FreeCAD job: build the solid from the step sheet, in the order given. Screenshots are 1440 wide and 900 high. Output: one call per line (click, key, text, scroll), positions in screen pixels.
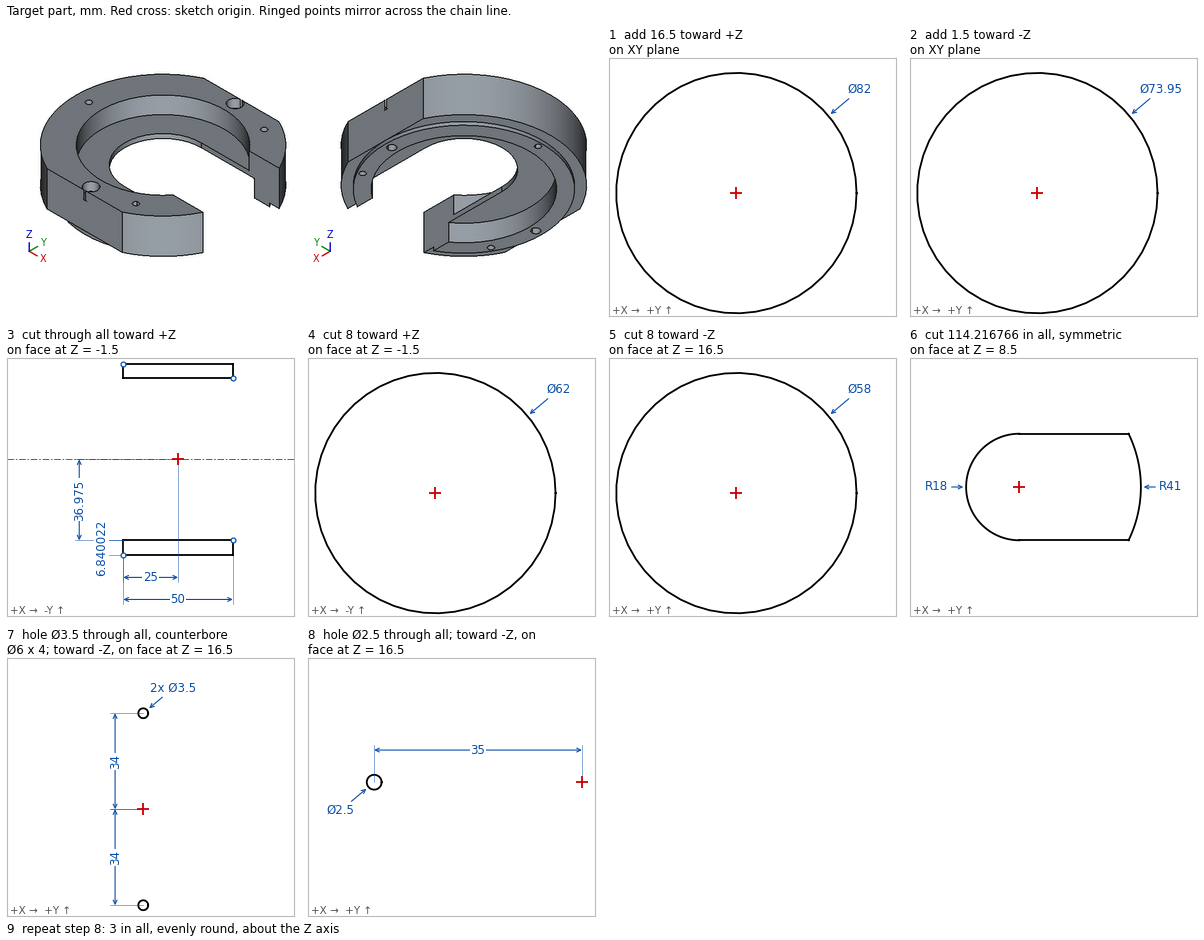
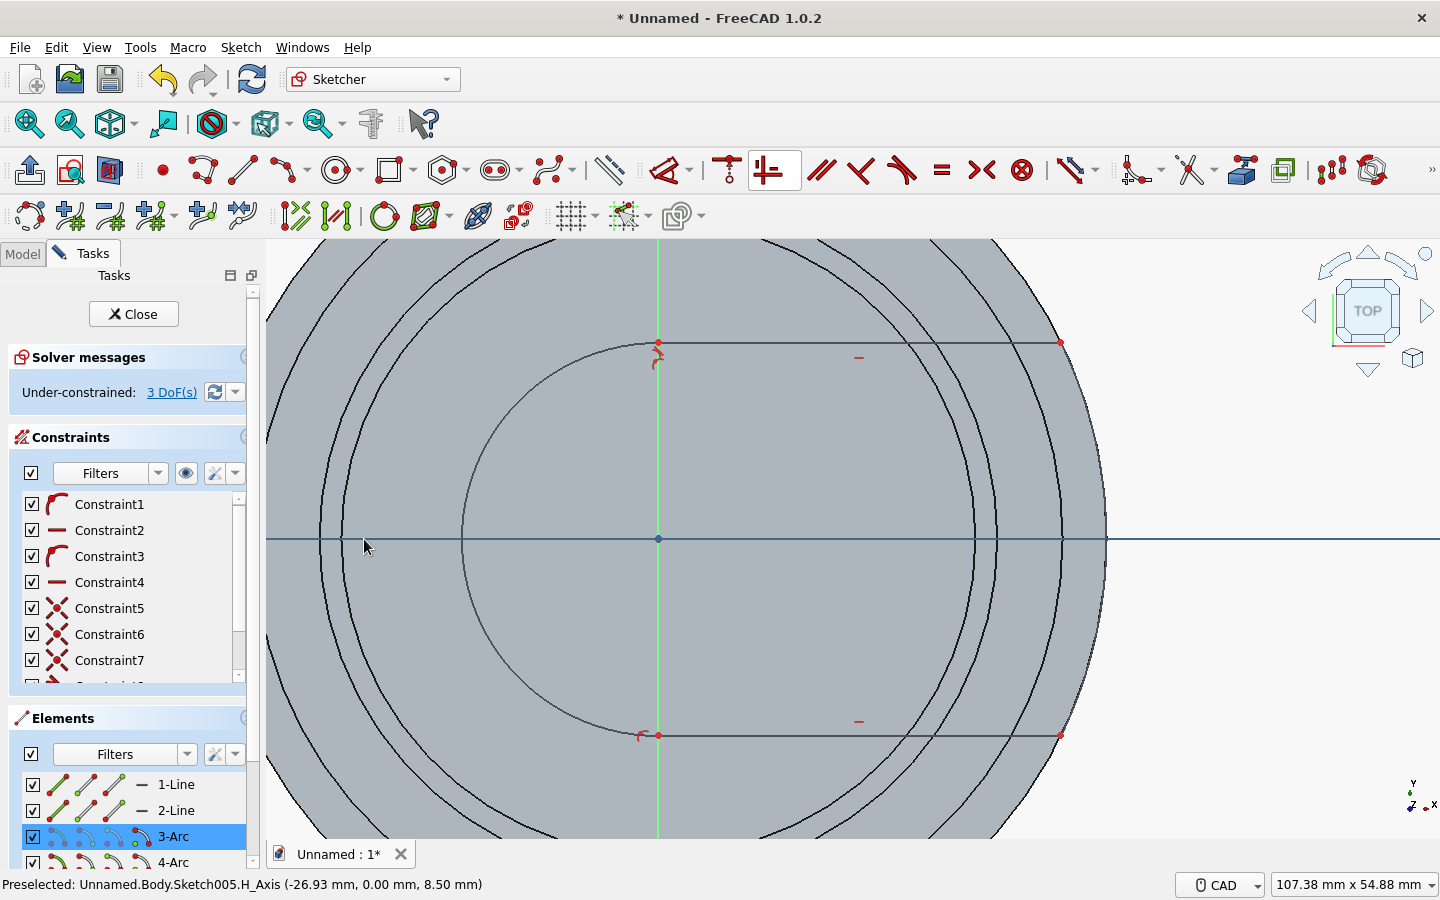
key(c)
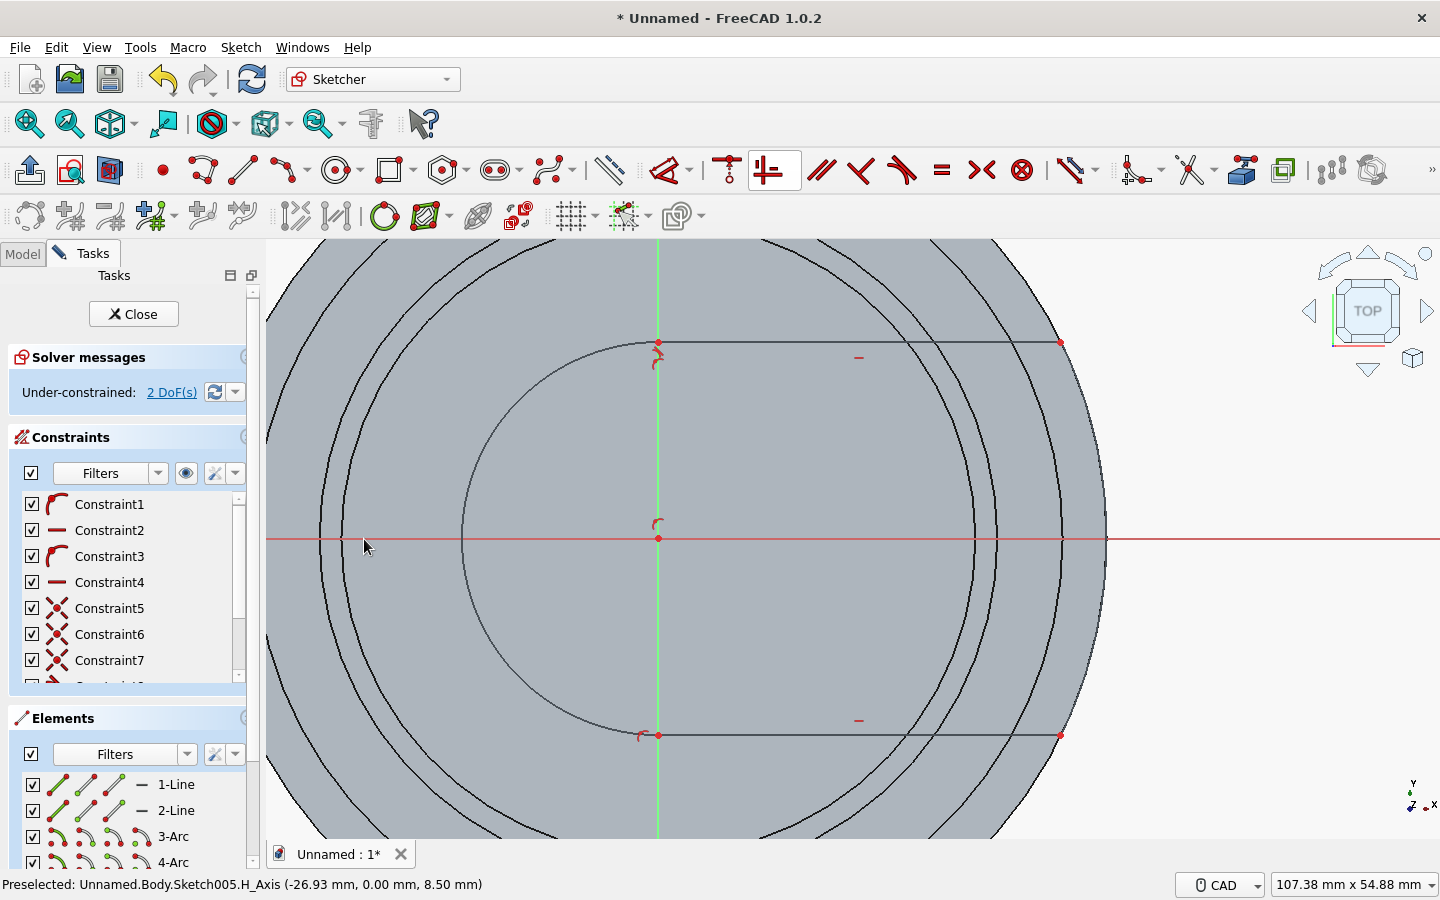
key(d)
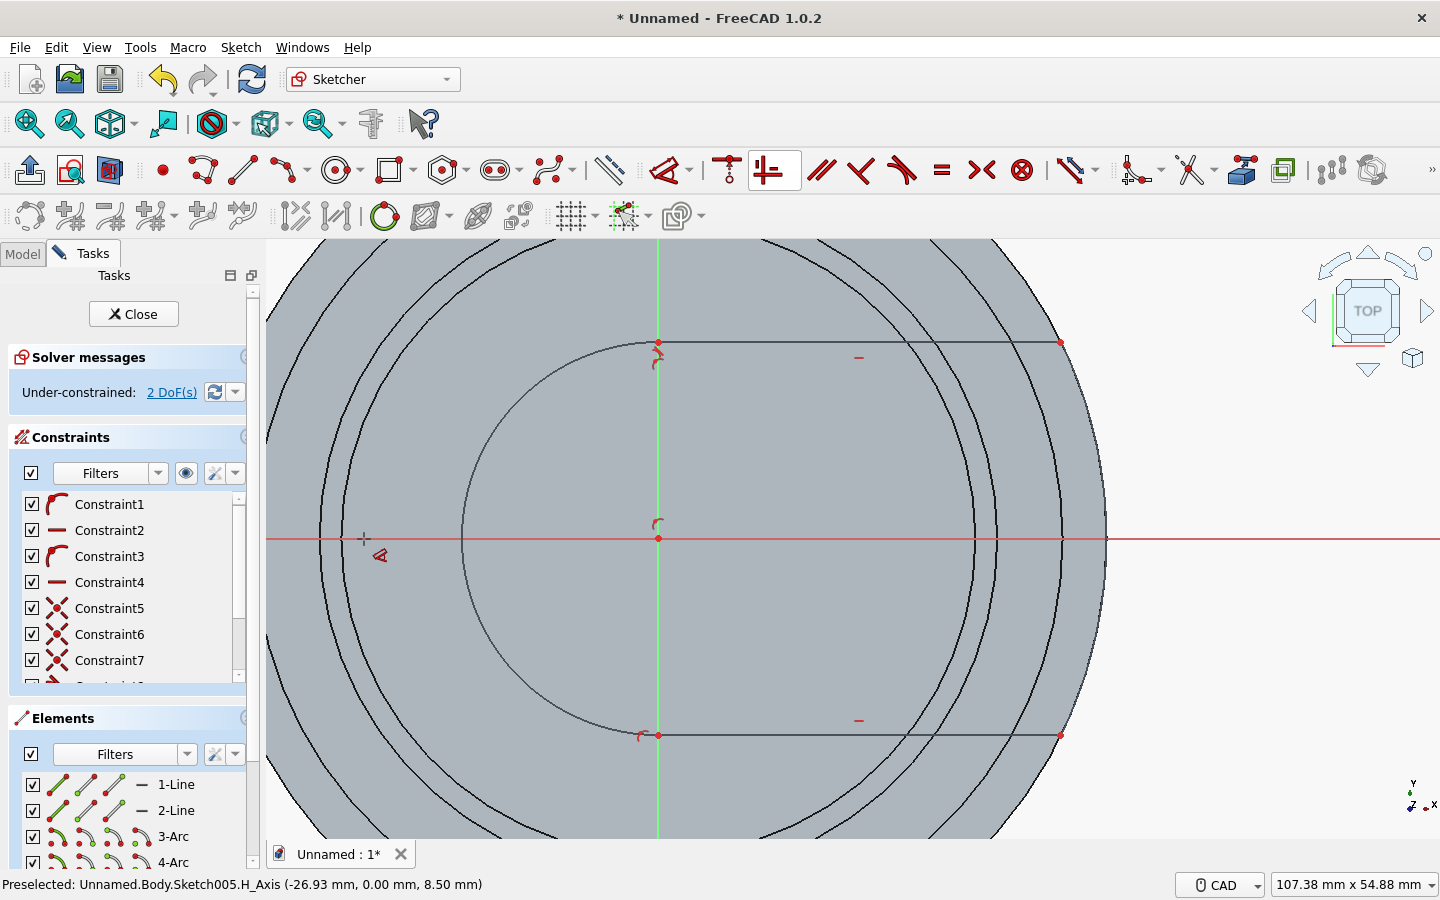
click(499, 423)
click(473, 404)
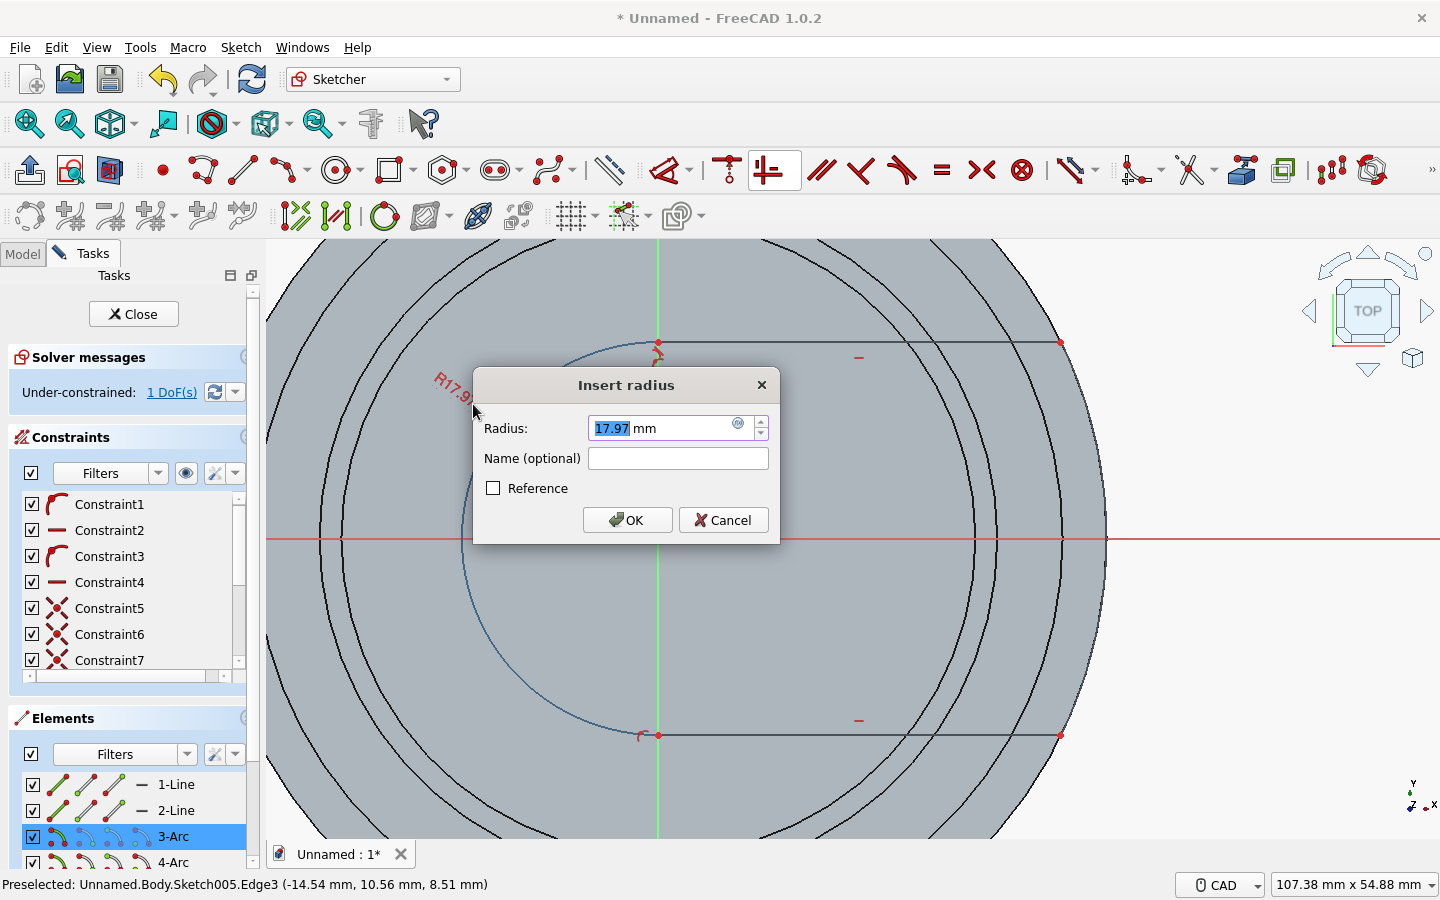
text(18)
key(Return)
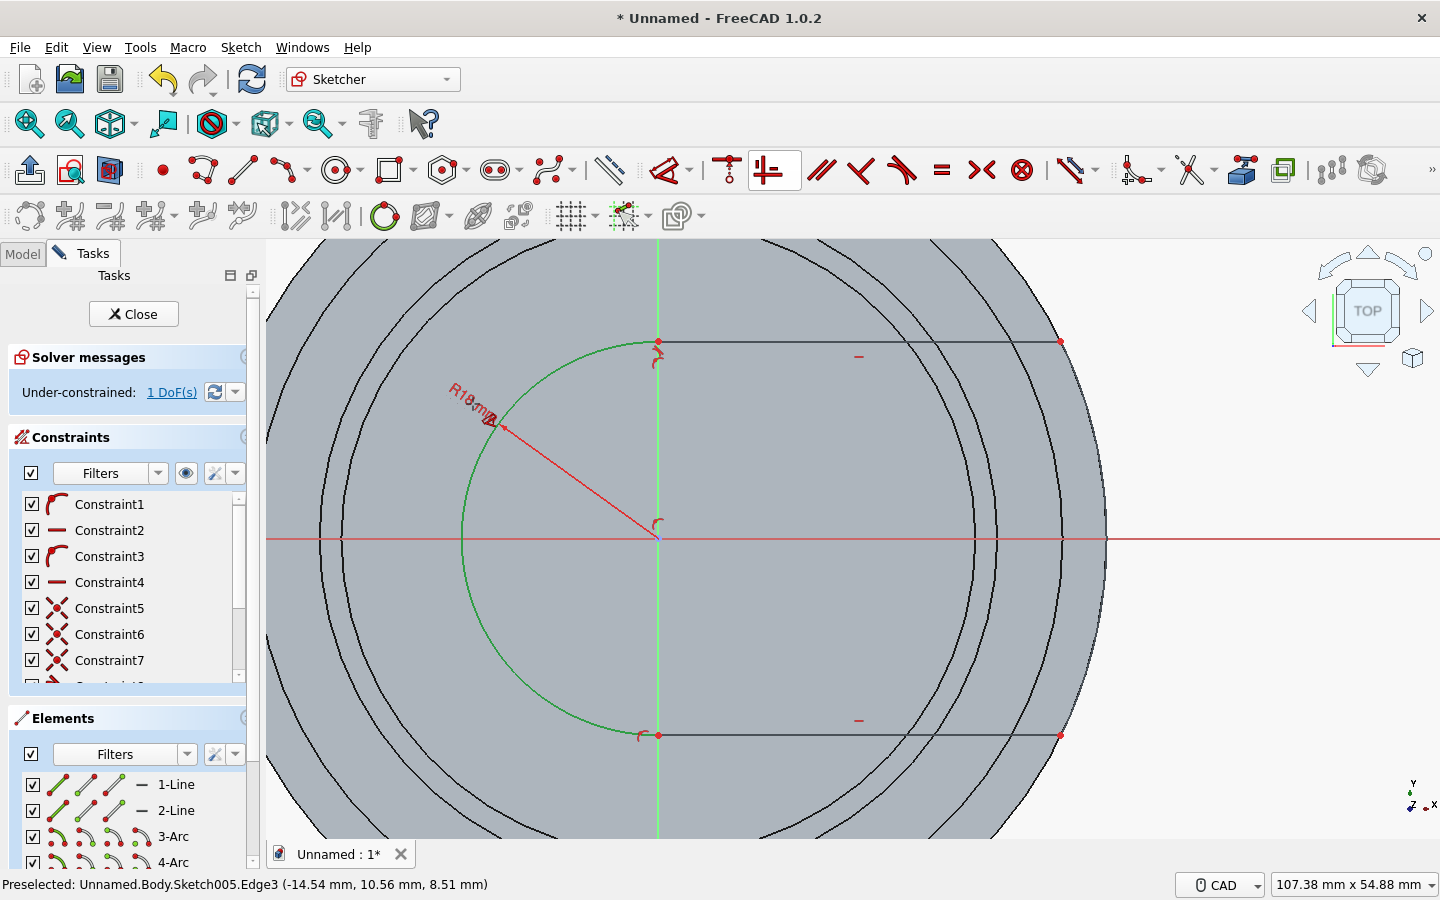
click(1099, 620)
click(1130, 626)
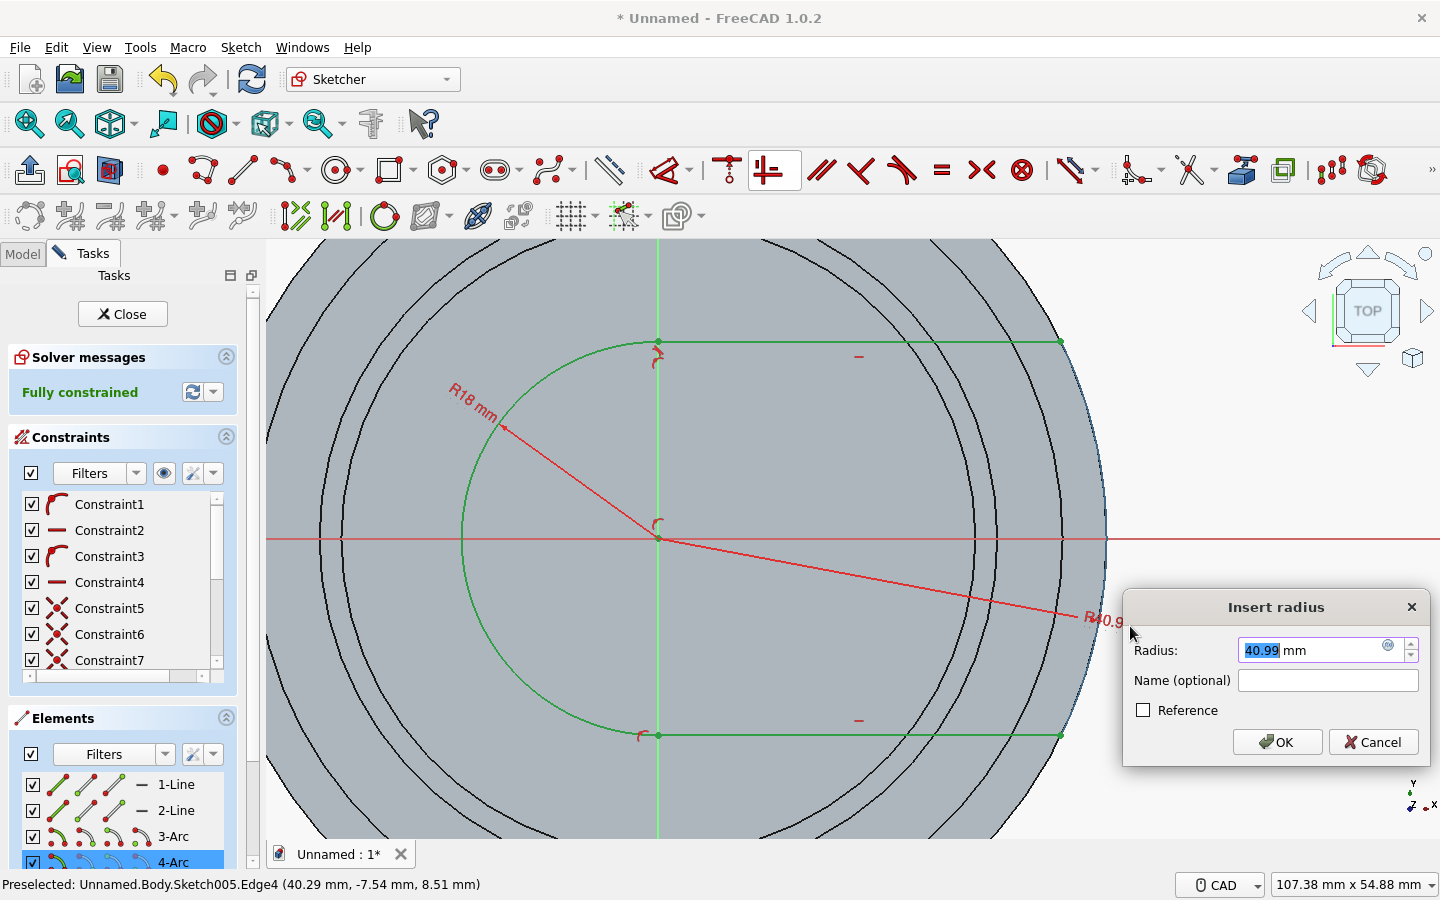
text(41)
key(Return)
key(Escape)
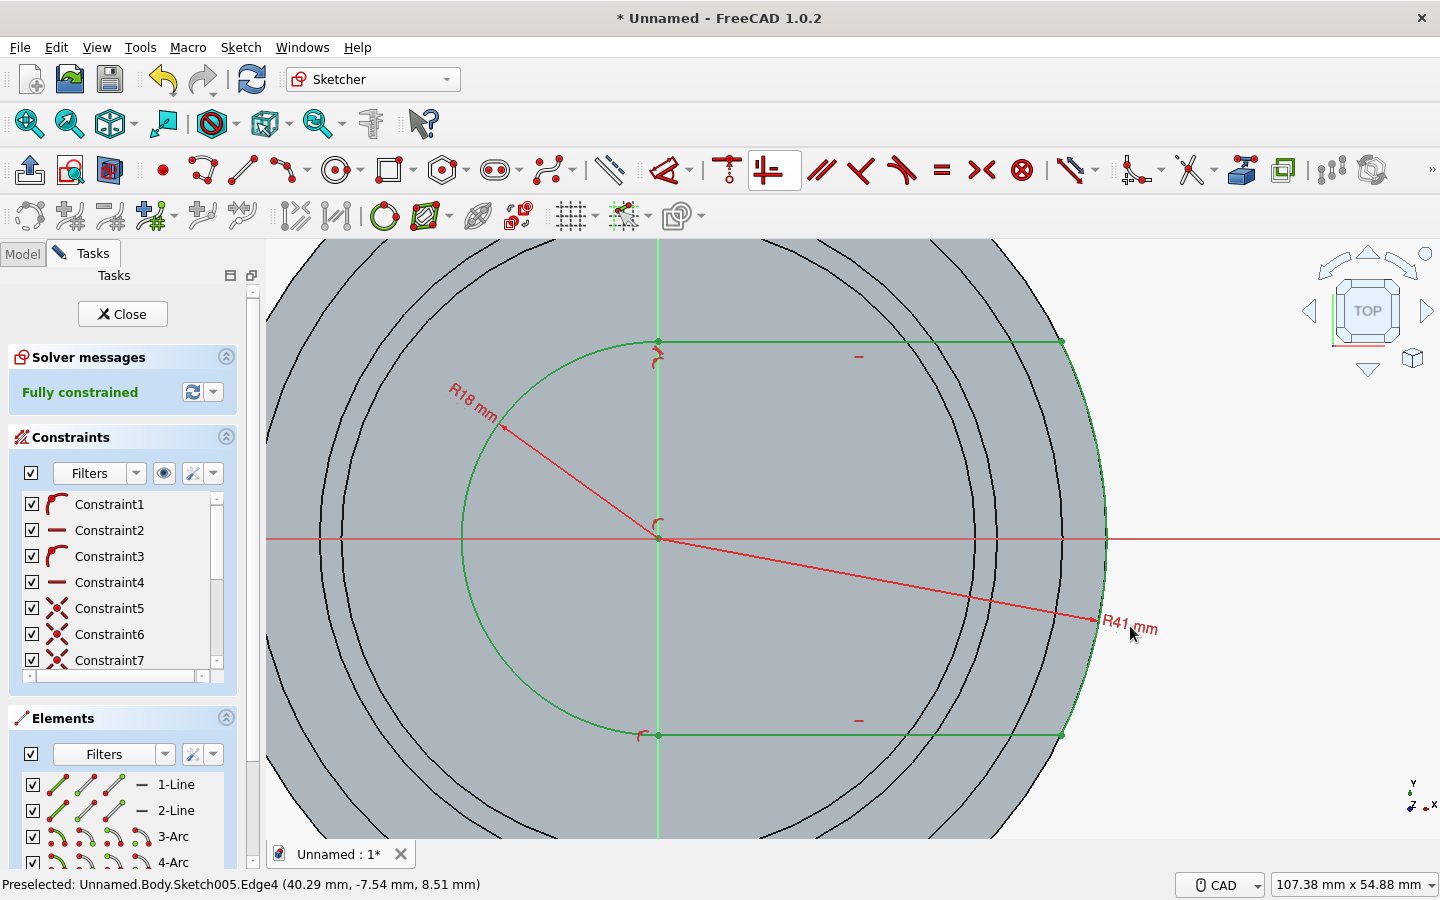
click(123, 314)